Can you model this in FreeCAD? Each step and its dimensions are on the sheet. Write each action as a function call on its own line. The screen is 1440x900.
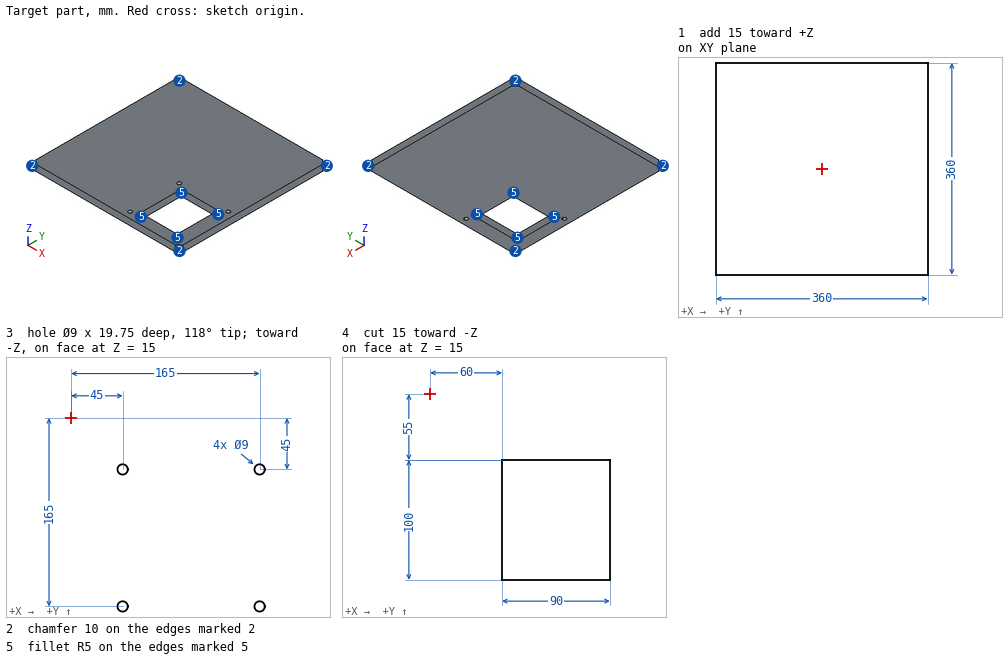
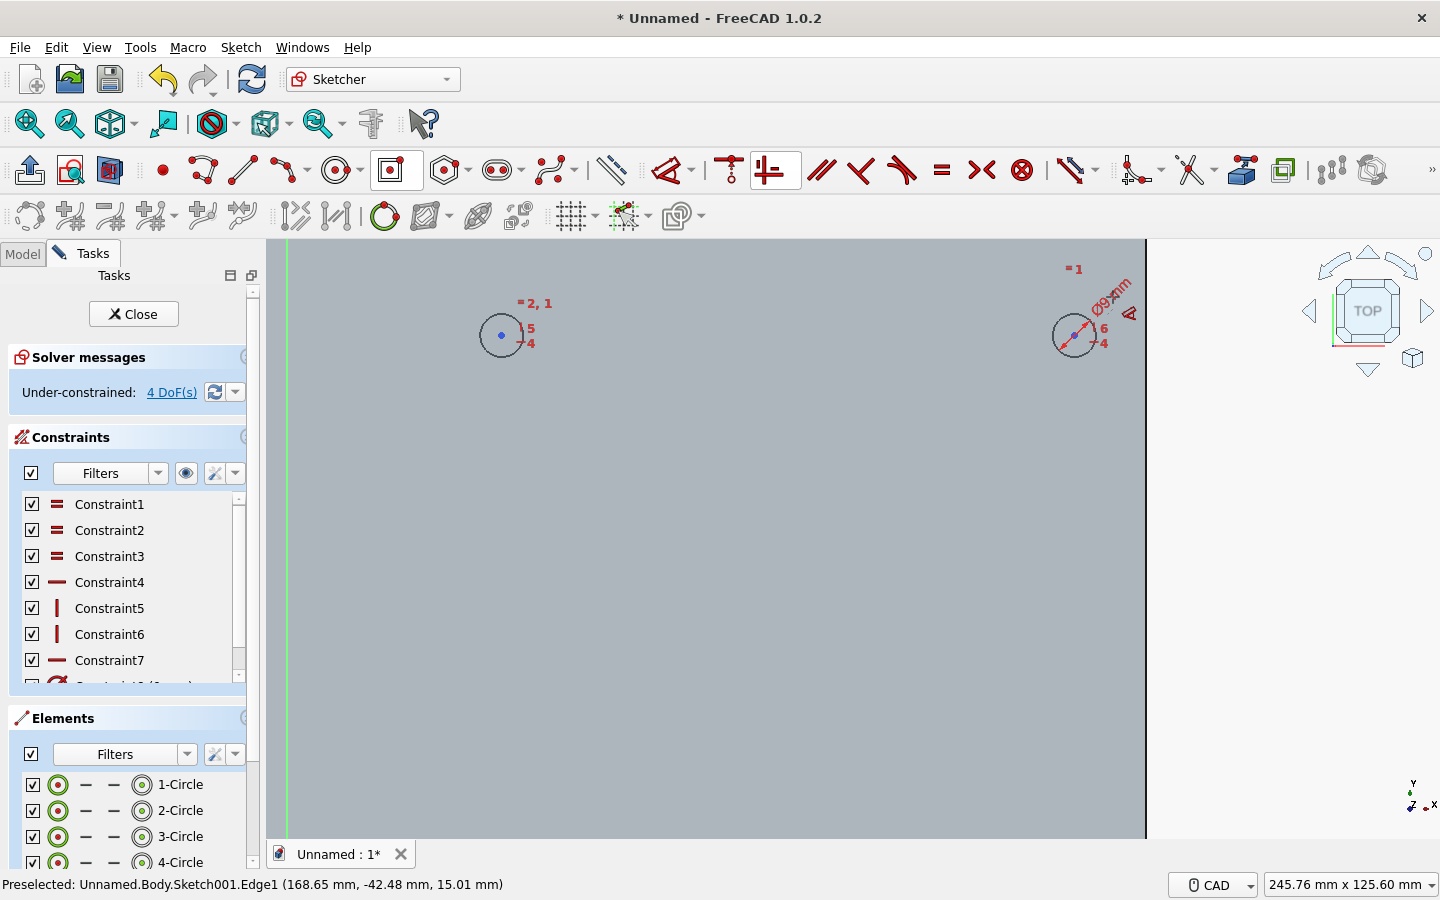
click(1074, 336)
click(1108, 277)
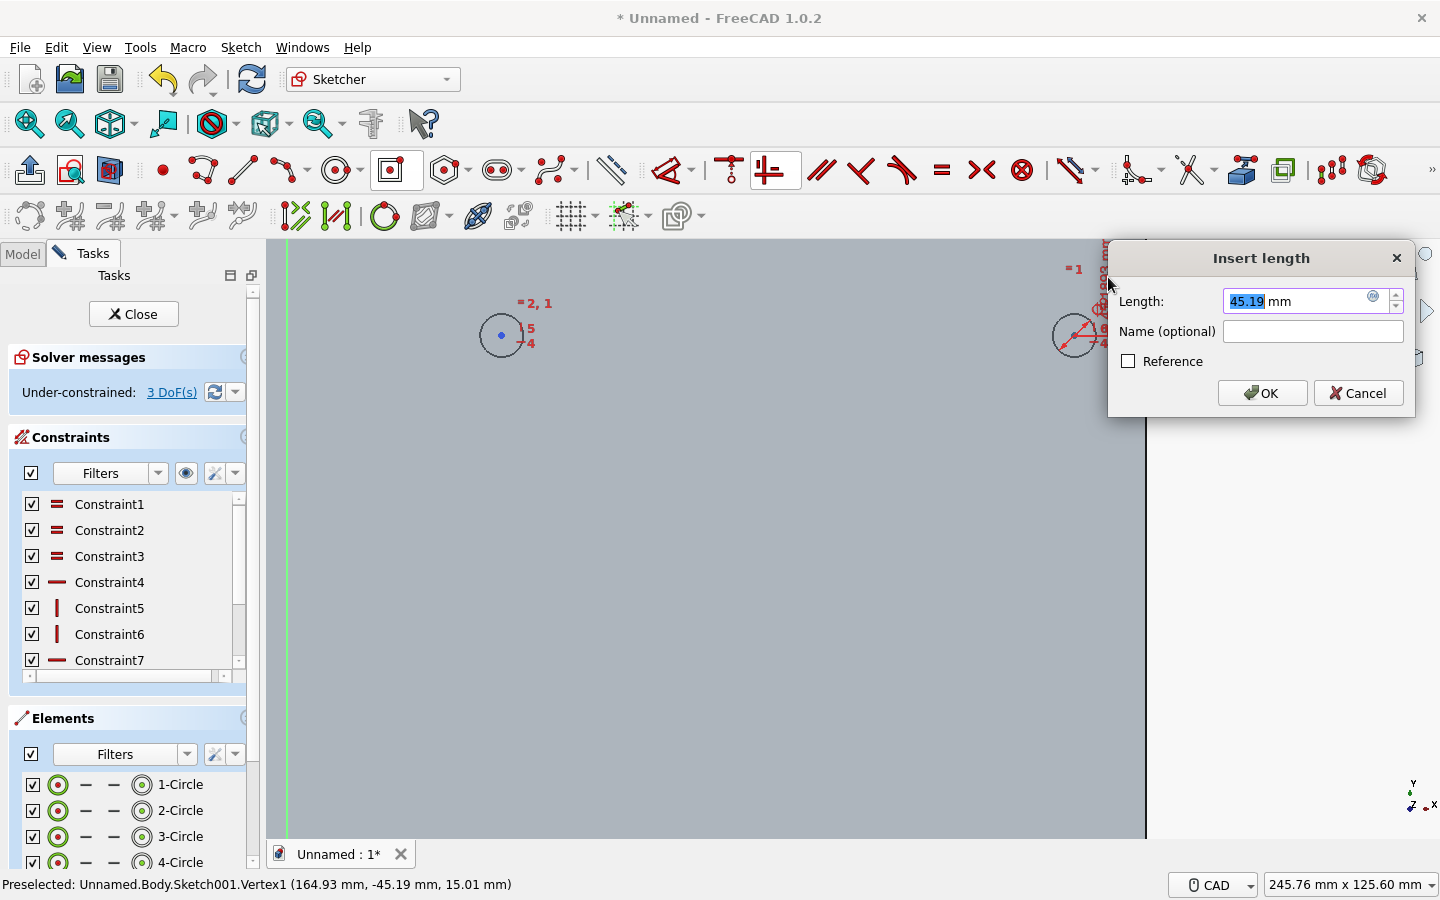
text(45)
key(Return)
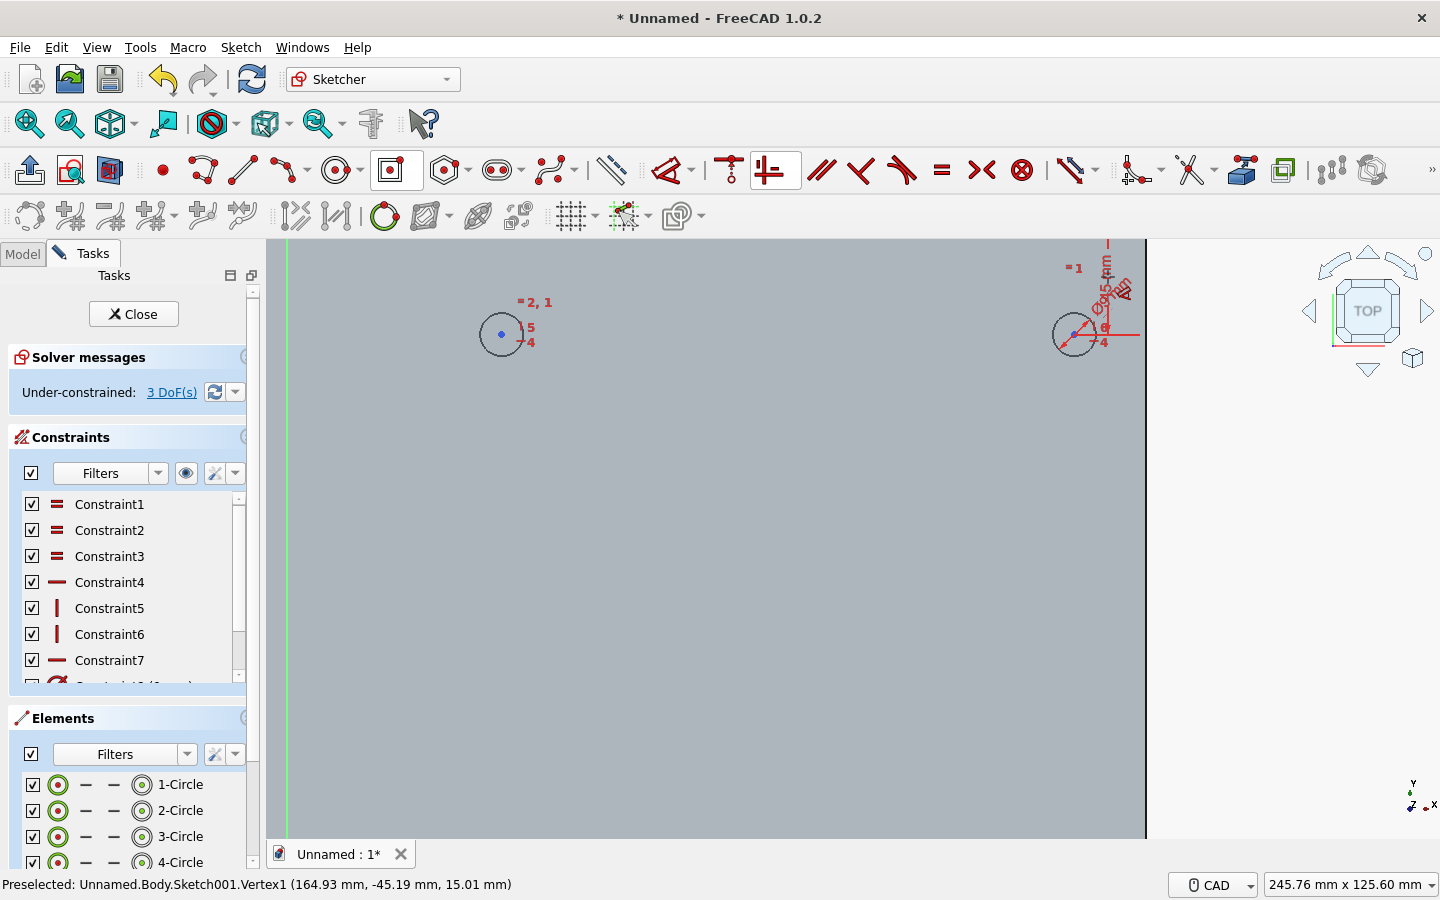
click(502, 335)
click(398, 369)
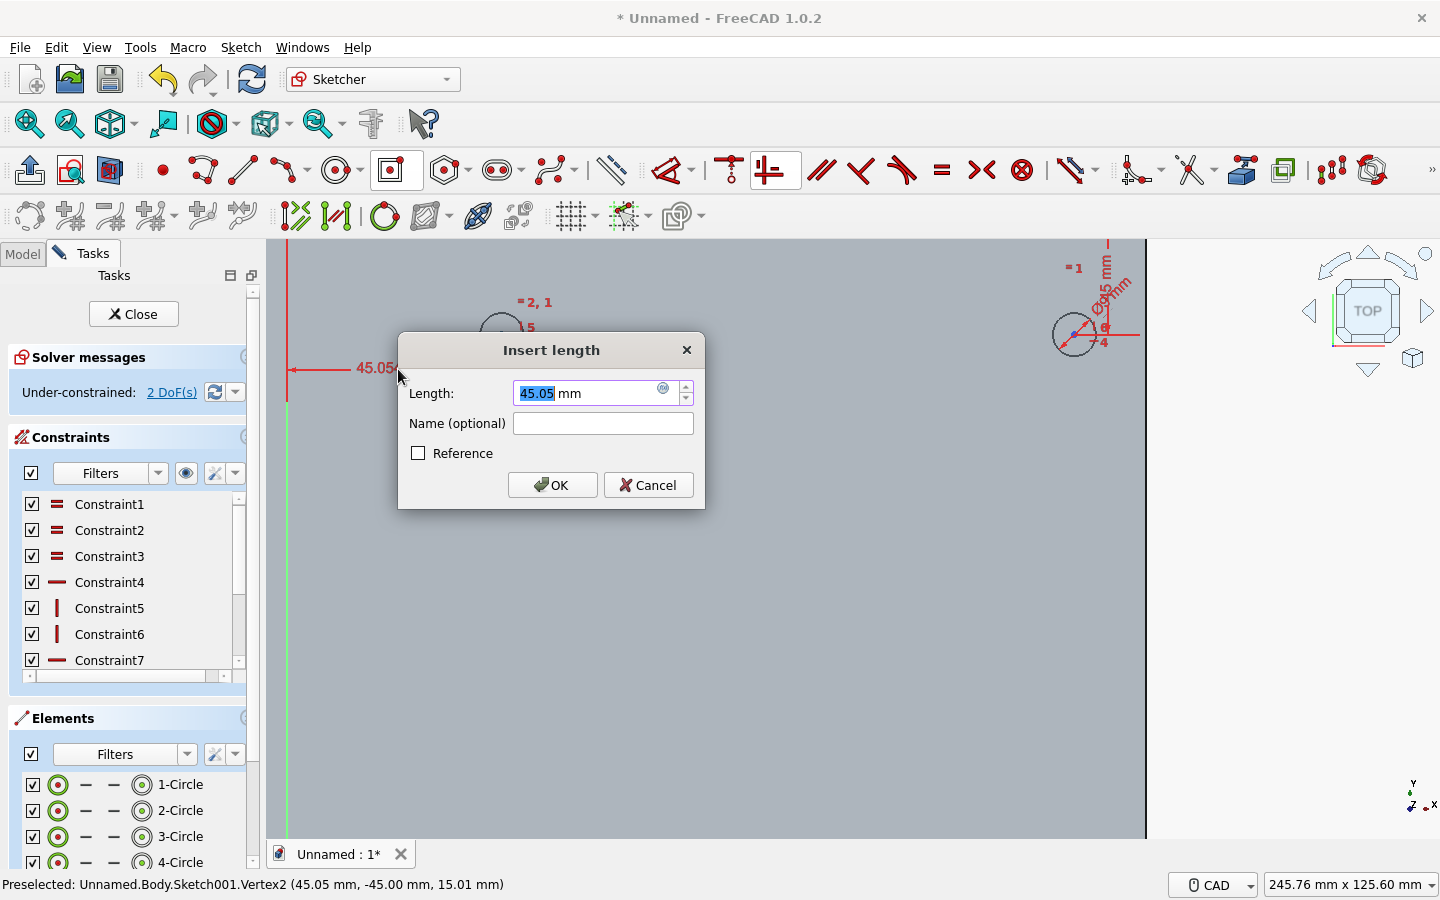
text(45)
key(Return)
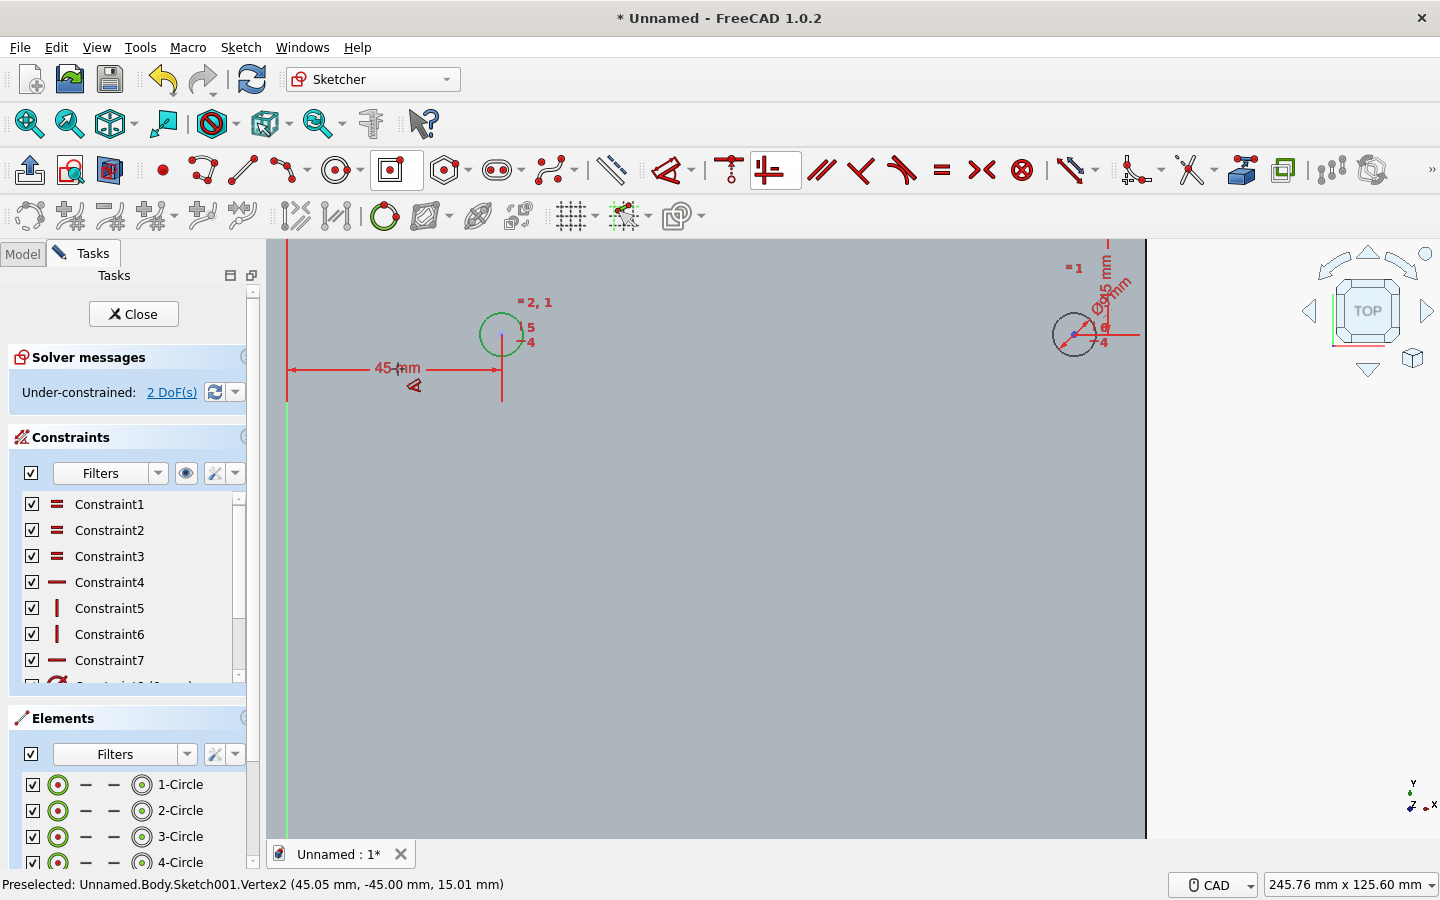
click(1074, 335)
click(684, 369)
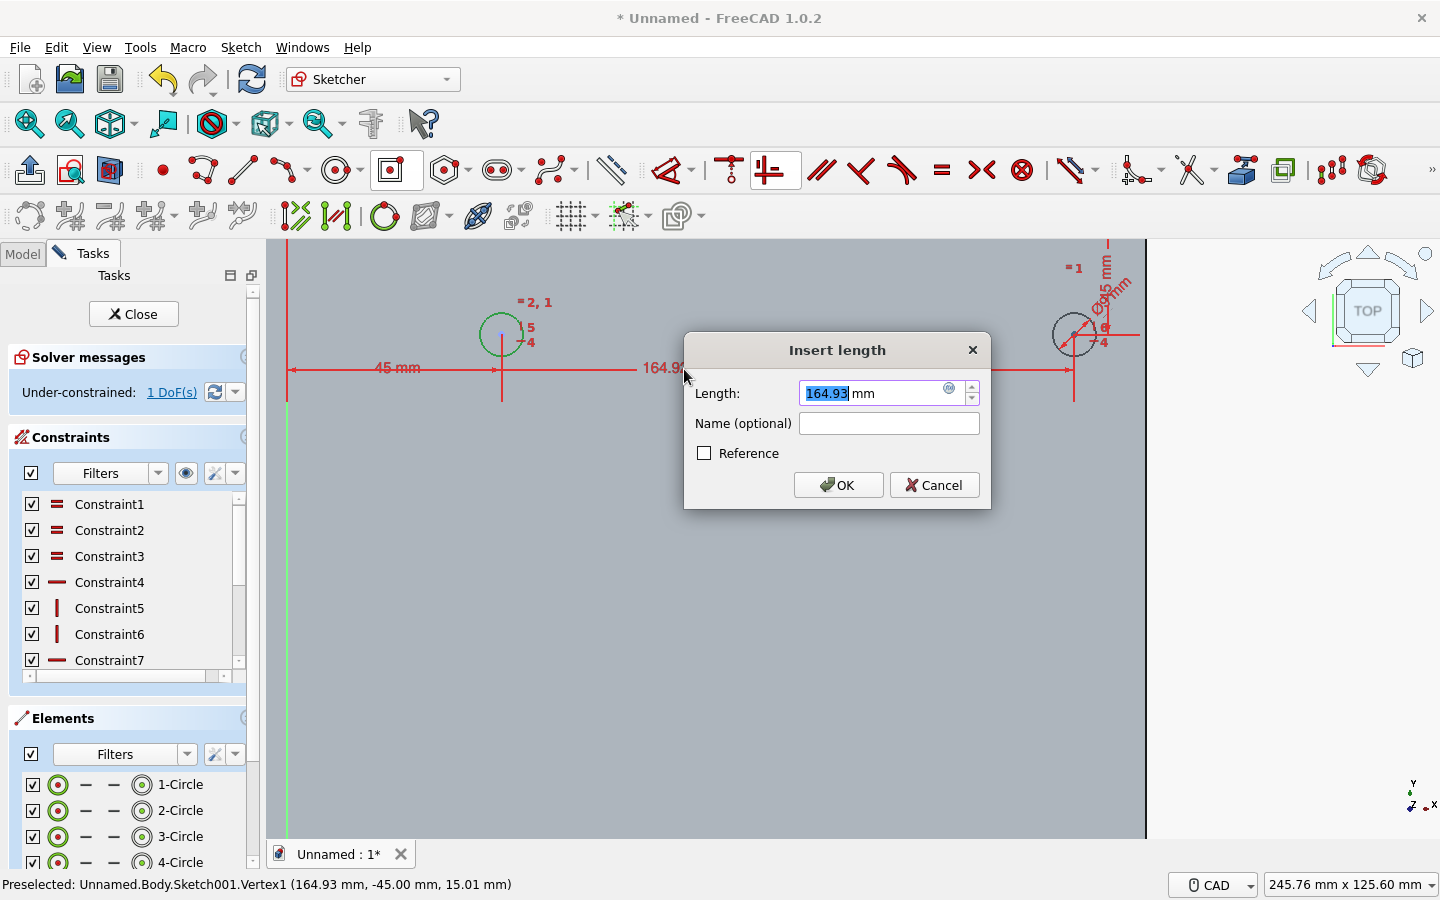
text(165)
key(Return)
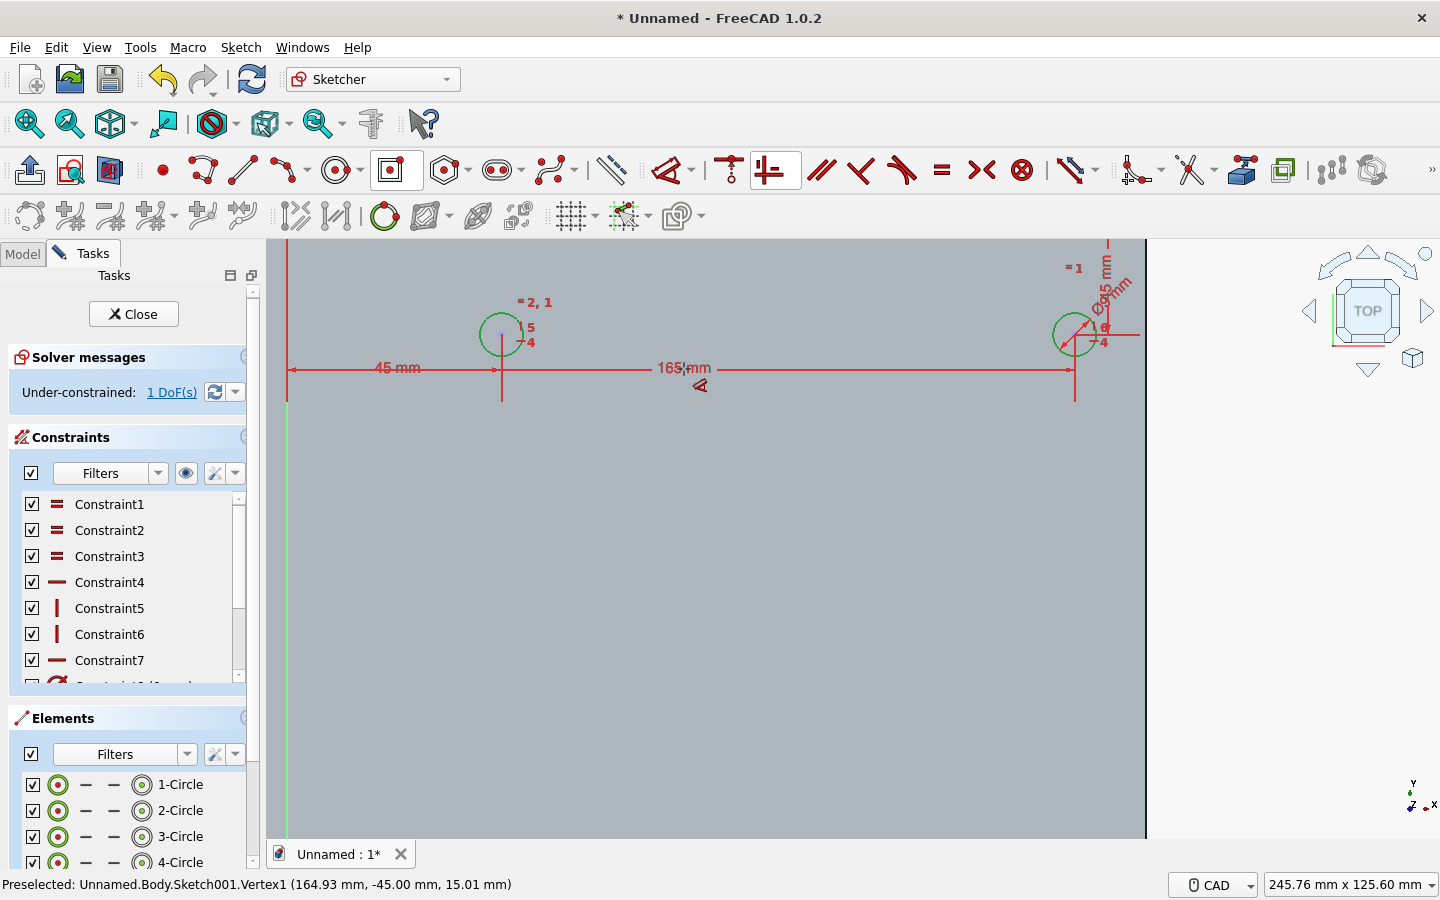
scroll(860, 551, down, 4)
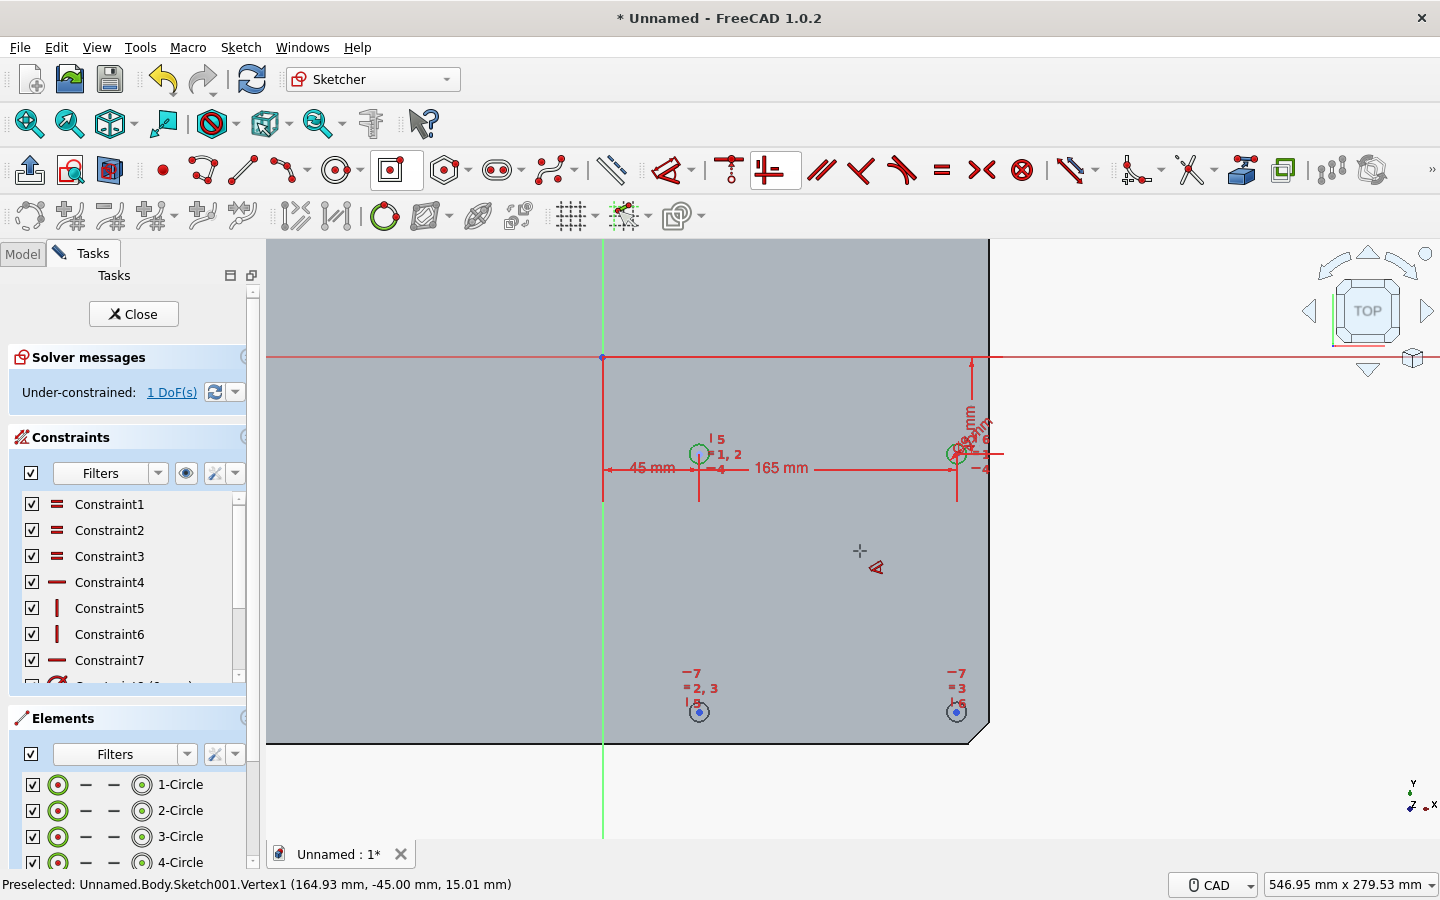
click(699, 712)
click(569, 535)